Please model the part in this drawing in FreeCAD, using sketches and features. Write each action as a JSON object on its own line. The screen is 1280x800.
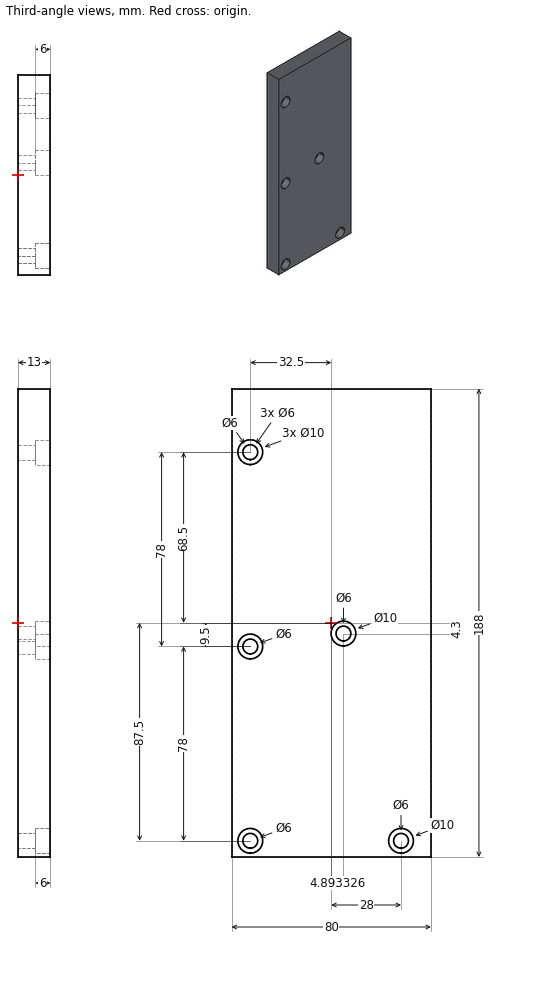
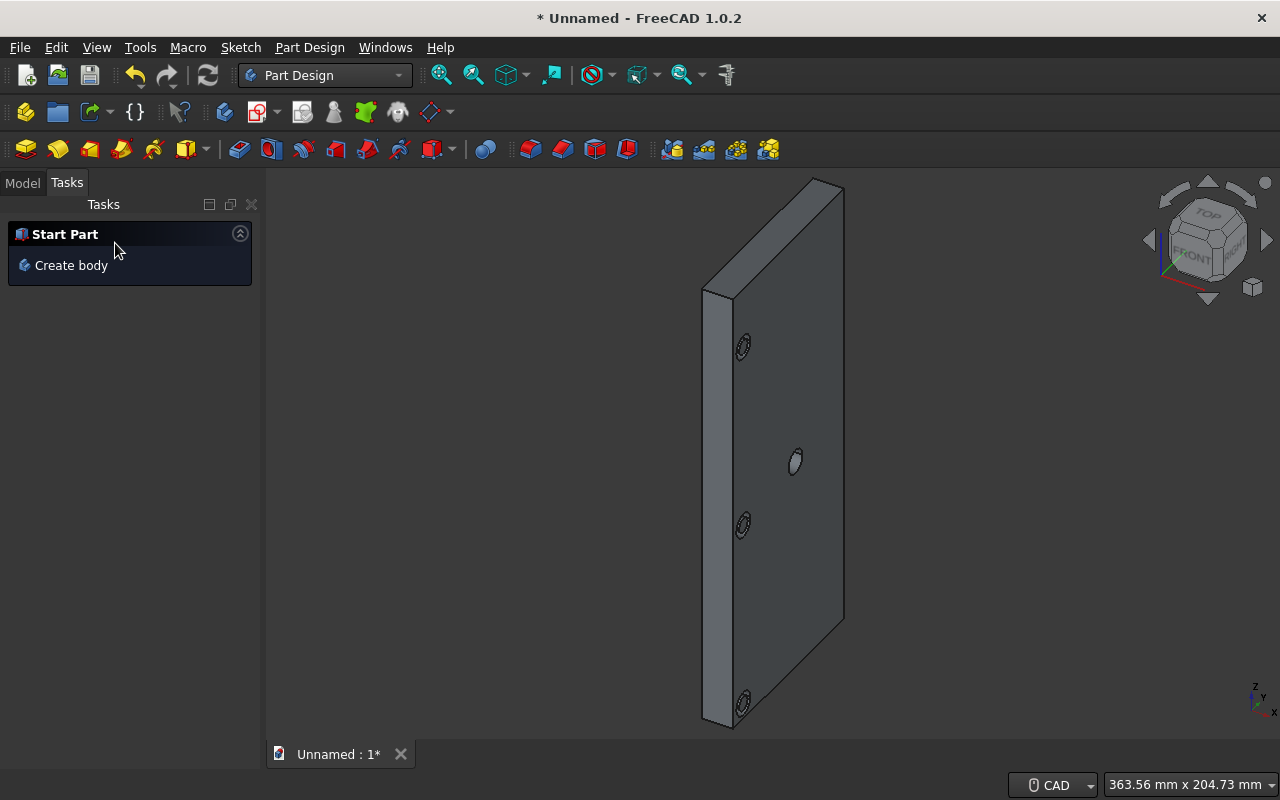
{"action": "left_click", "coordinate": [789, 580]}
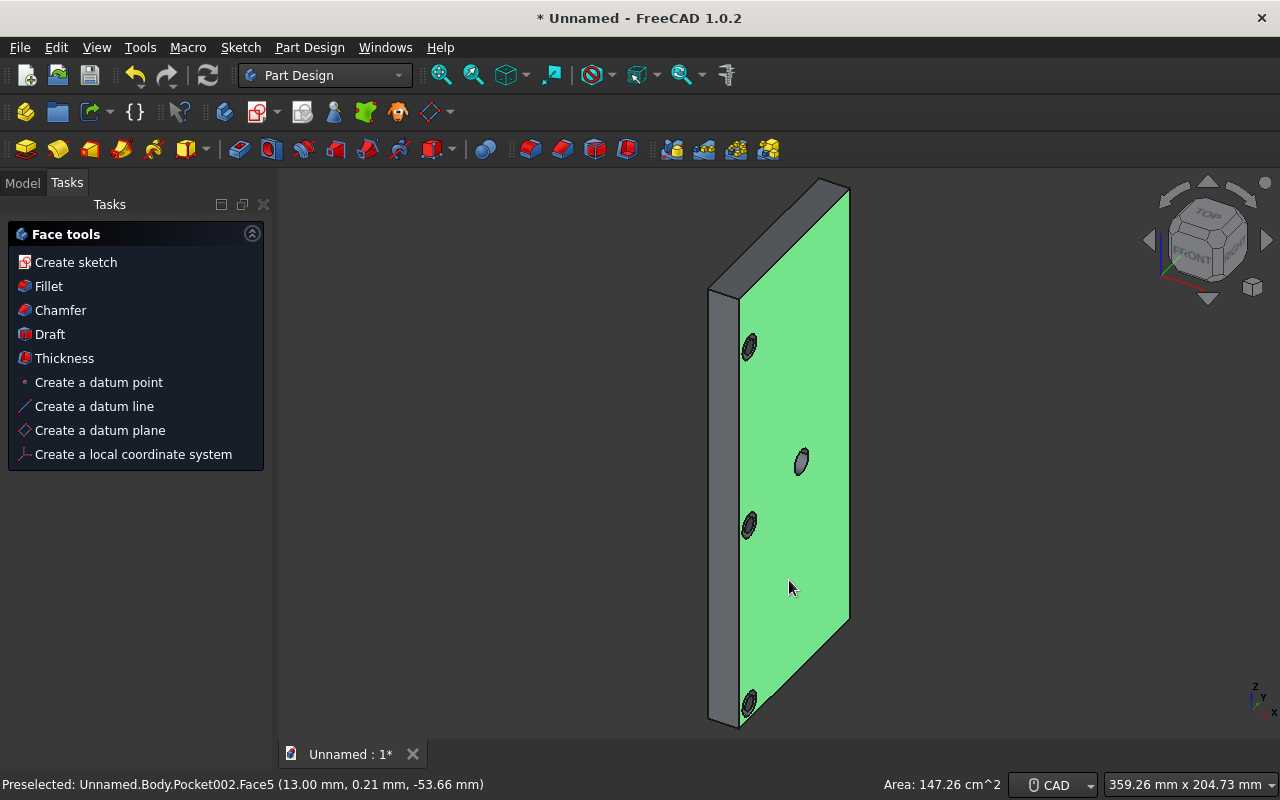
{"action": "left_click", "coordinate": [258, 112]}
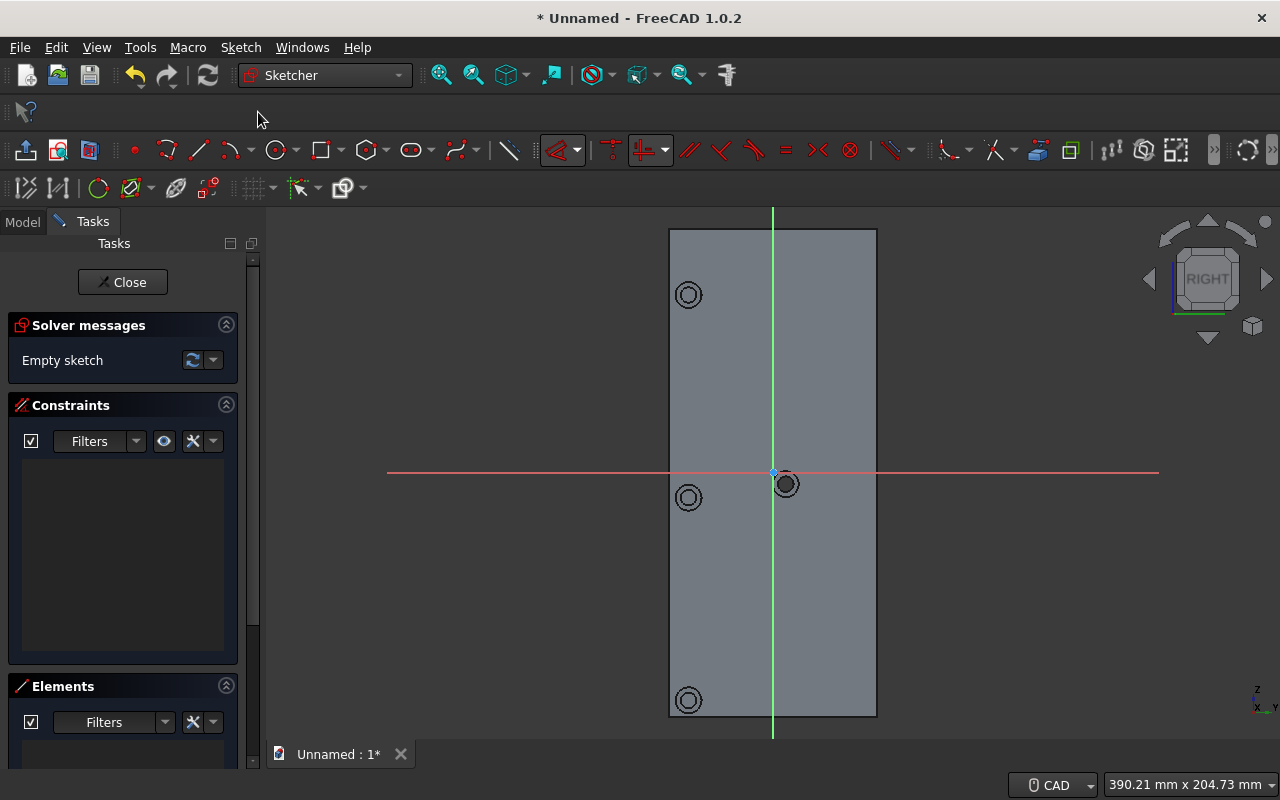
{"action": "scroll", "coordinate": [688, 286], "scroll_direction": "up", "scroll_amount": 15}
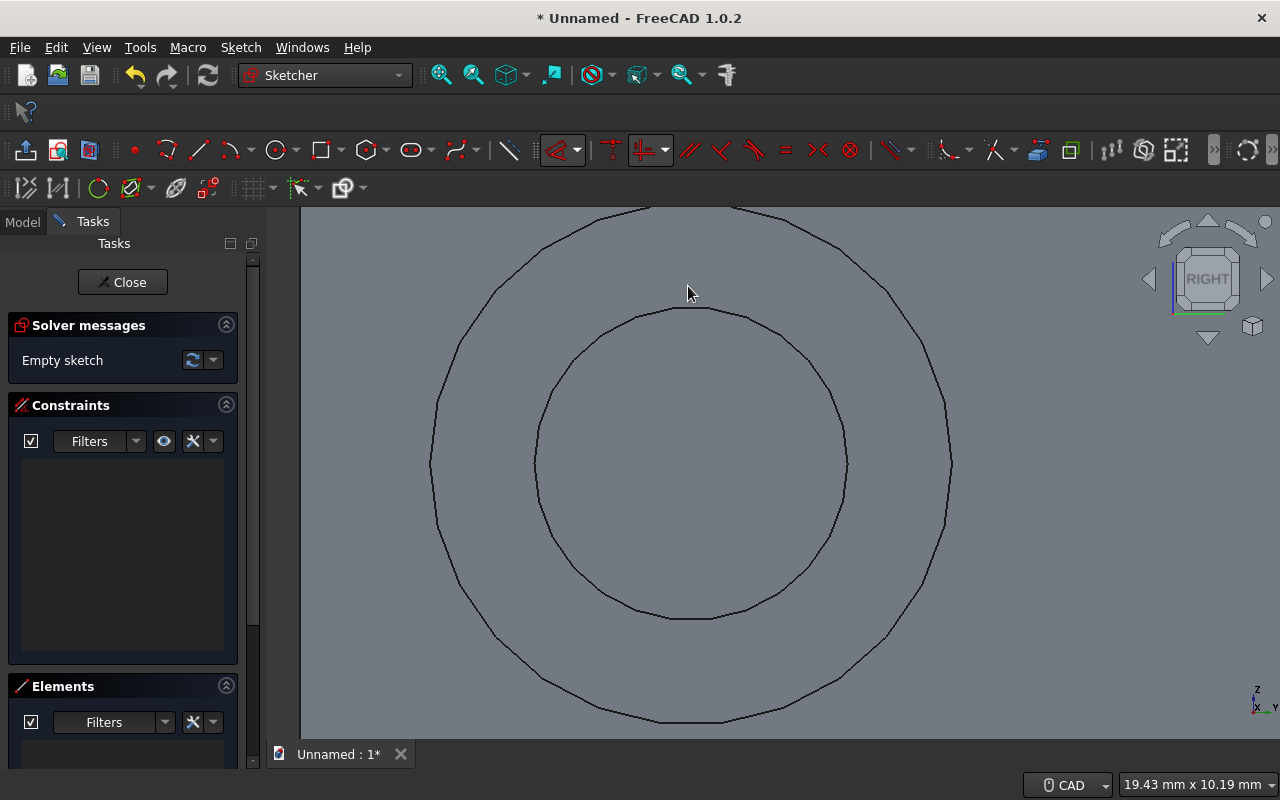
{"action": "left_click", "coordinate": [276, 150]}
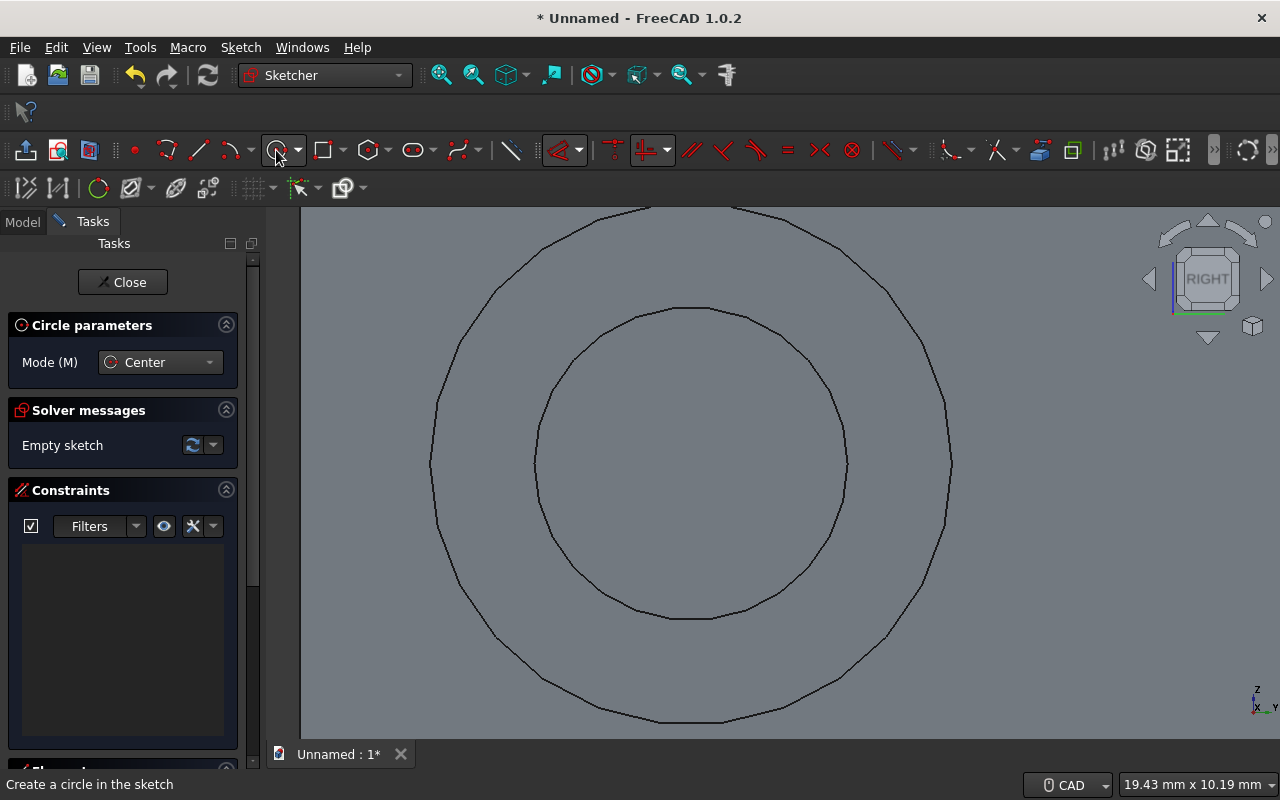
{"action": "left_click", "coordinate": [691, 464]}
{"action": "left_click", "coordinate": [802, 353]}
{"action": "key", "text": "Escape"}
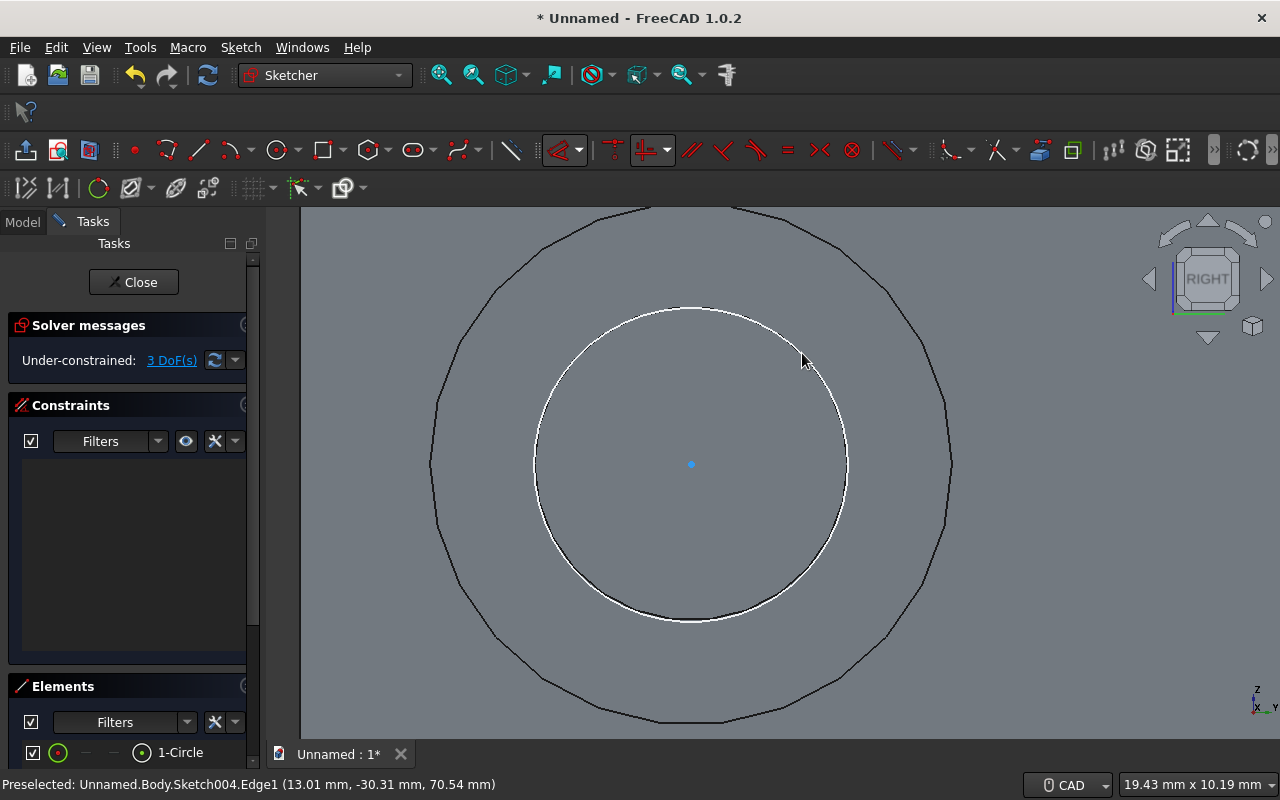
{"action": "left_click", "coordinate": [802, 354]}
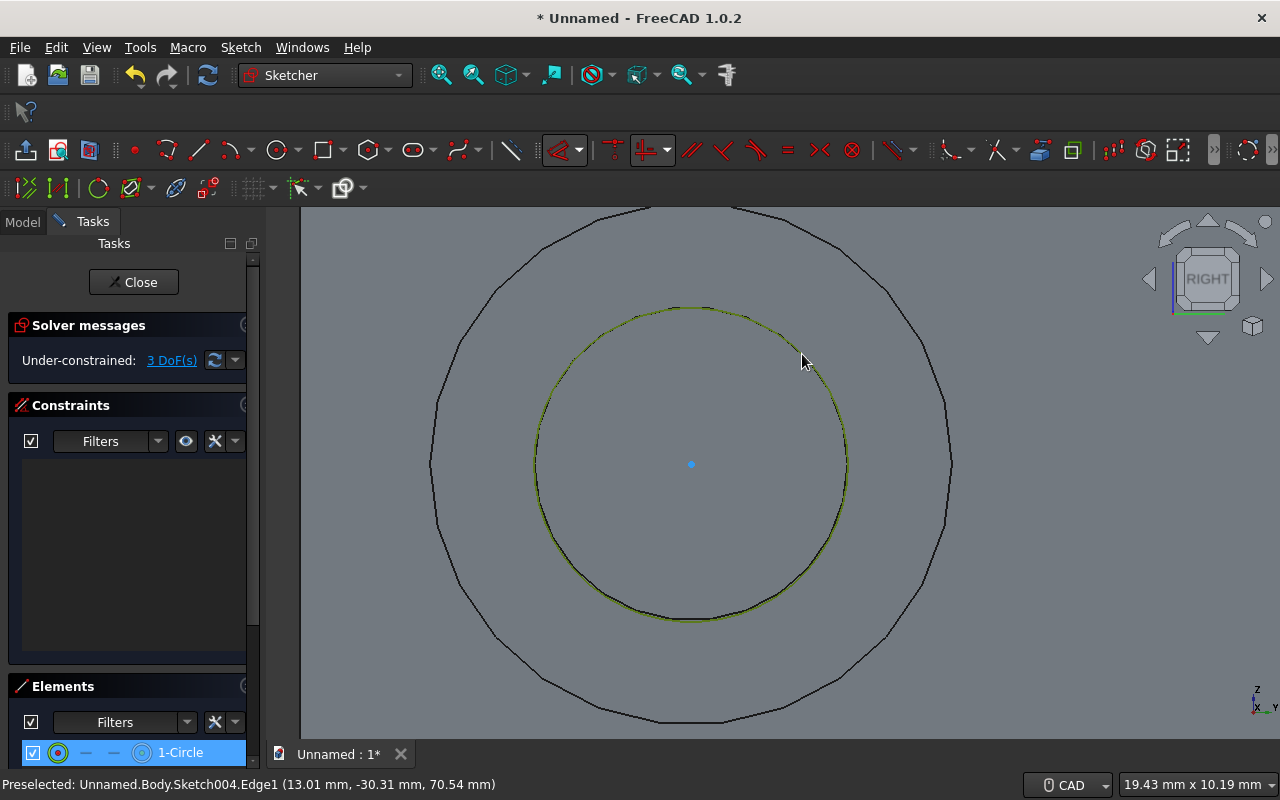
{"action": "key", "text": "k o"}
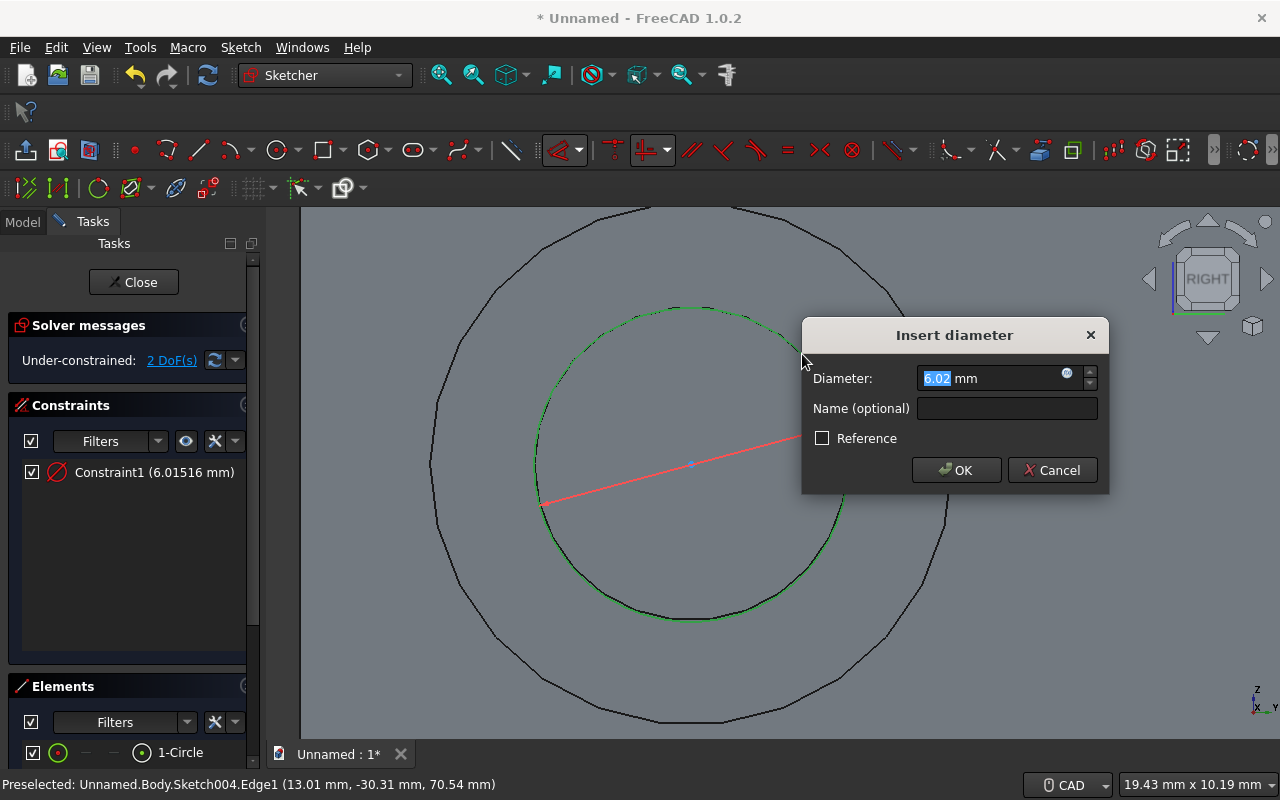
{"action": "type", "text": "6"}
{"action": "key", "text": "Return"}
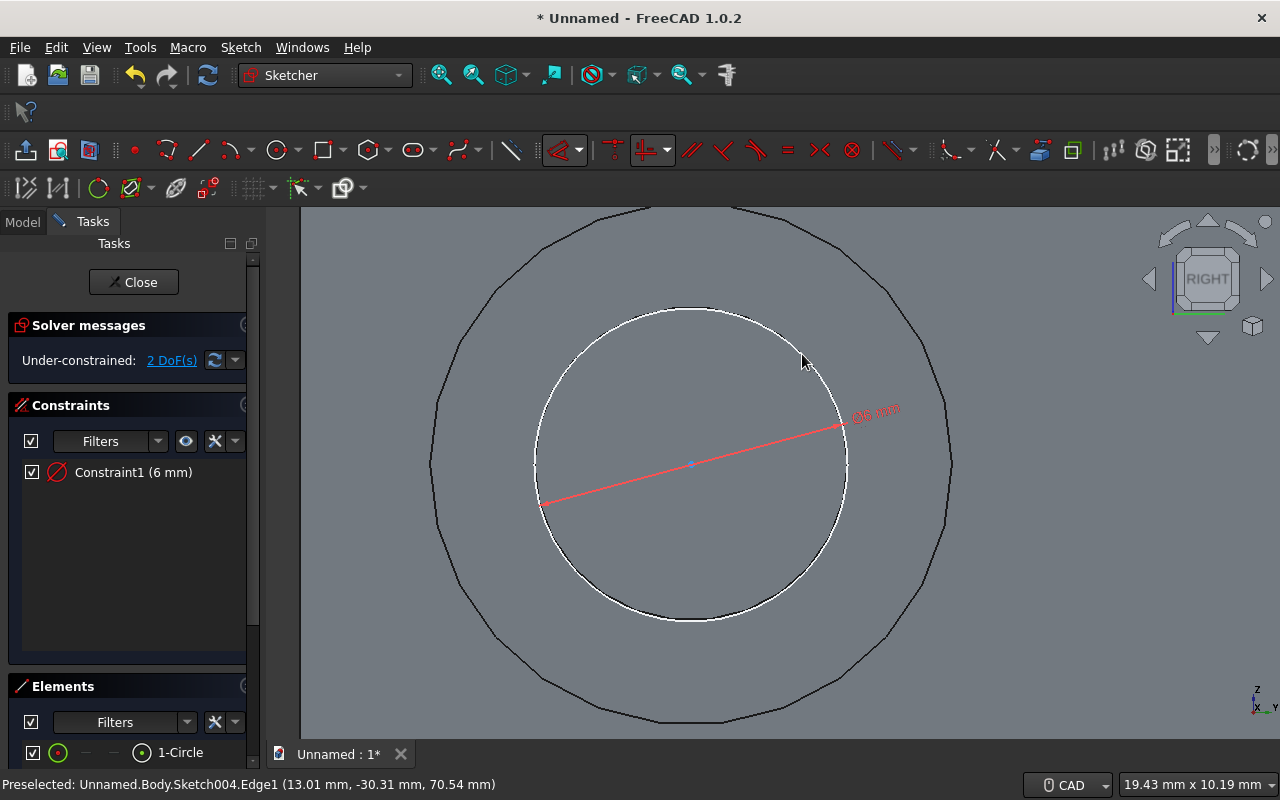
{"action": "left_click", "coordinate": [691, 465]}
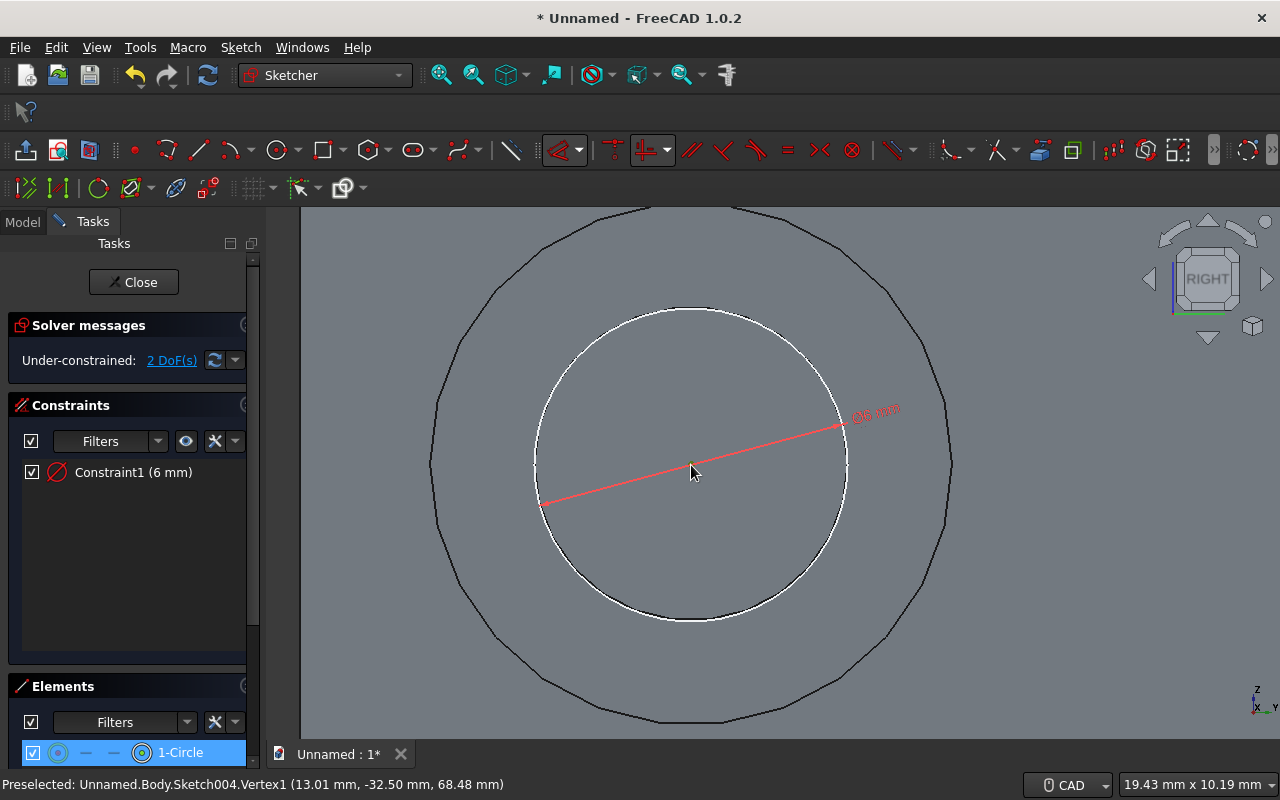
{"action": "left_click", "coordinate": [582, 150]}